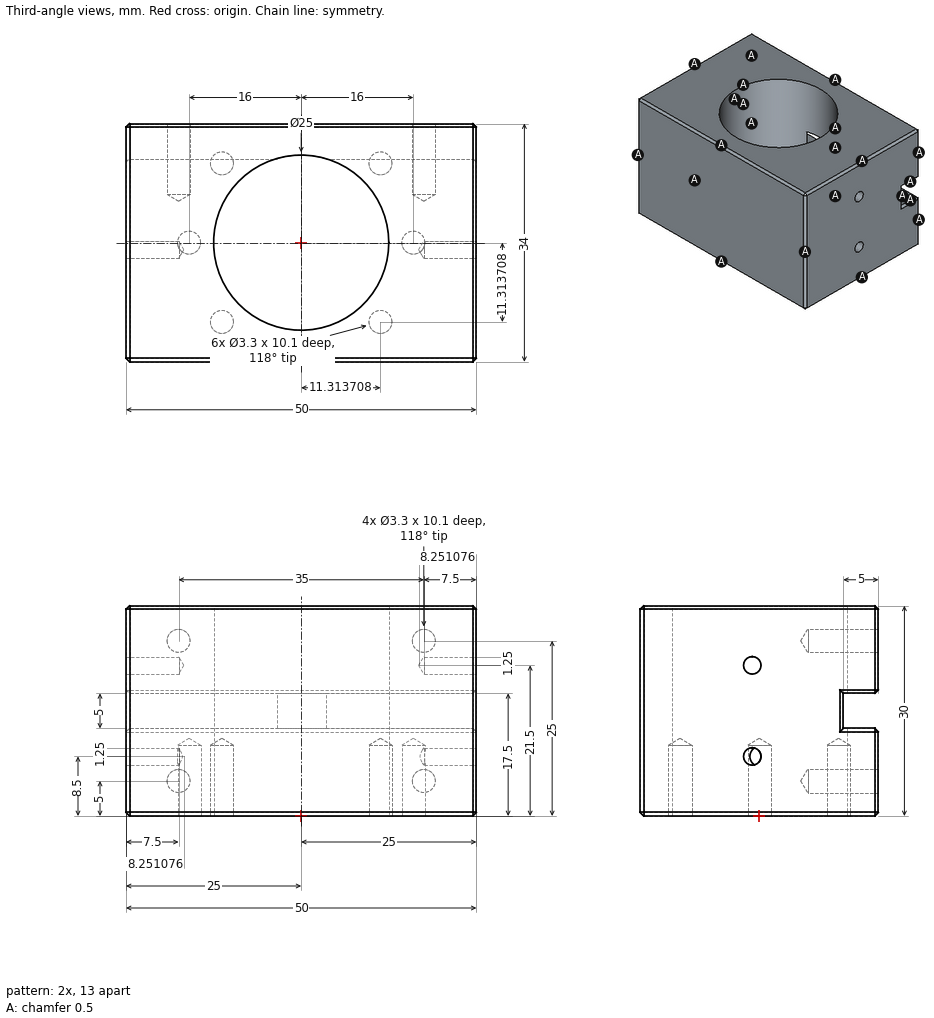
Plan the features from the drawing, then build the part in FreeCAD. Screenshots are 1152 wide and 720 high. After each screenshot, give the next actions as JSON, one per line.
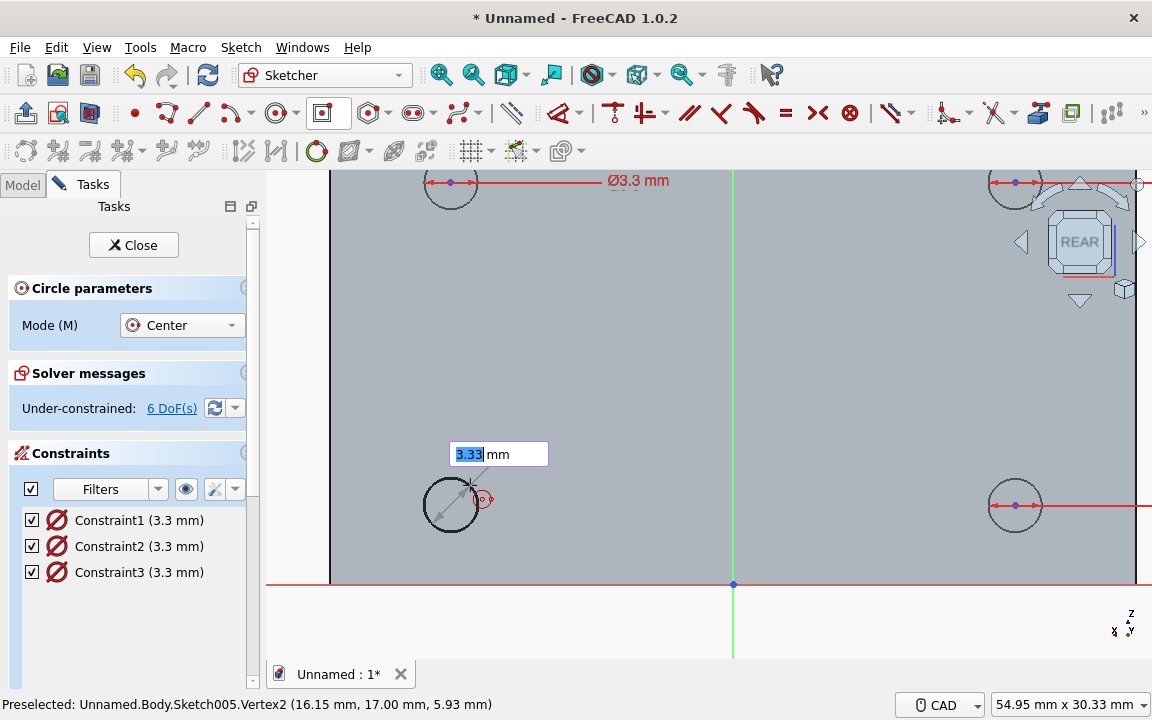
{"action": "type", "text": "3.3"}
{"action": "key", "text": "Return"}
{"action": "key", "text": "Escape"}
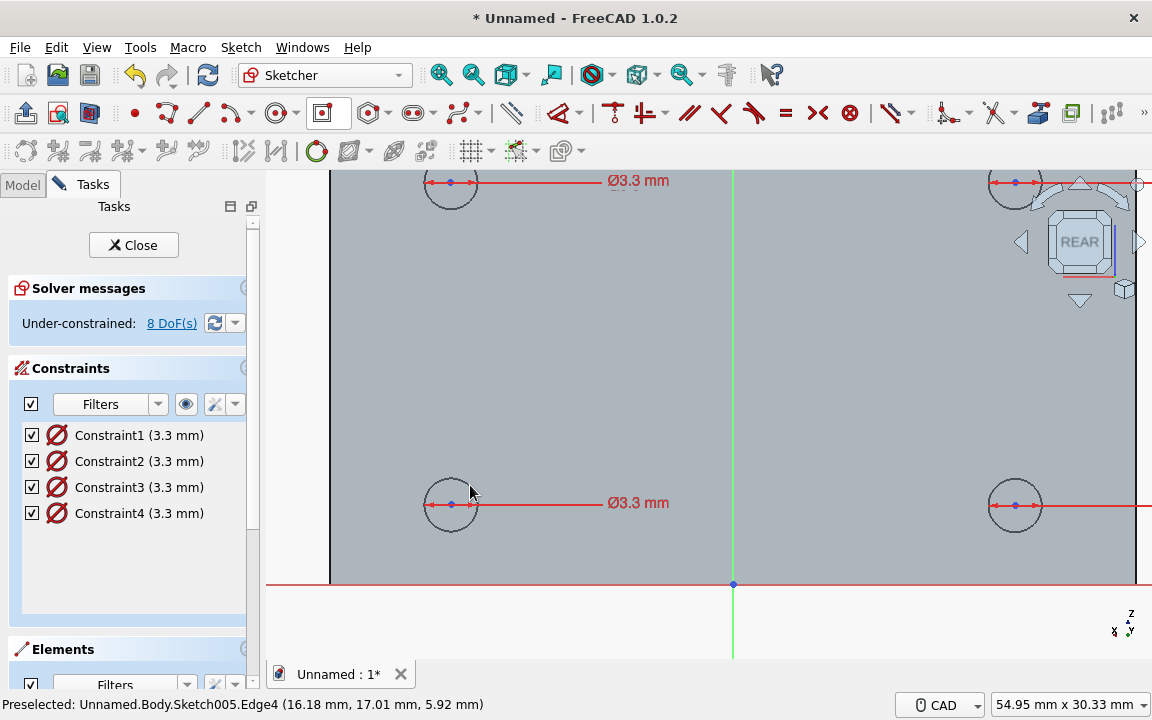
{"action": "scroll", "coordinate": [452, 505], "scroll_direction": "down", "scroll_amount": 2}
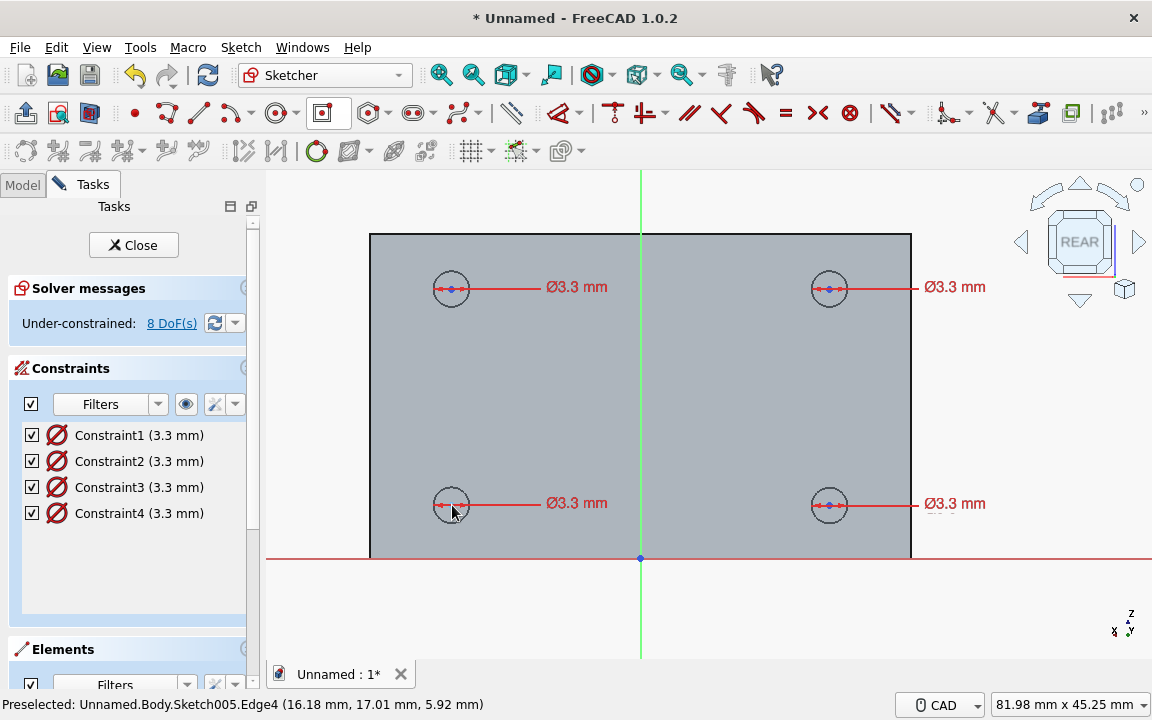
{"action": "left_click", "coordinate": [451, 289]}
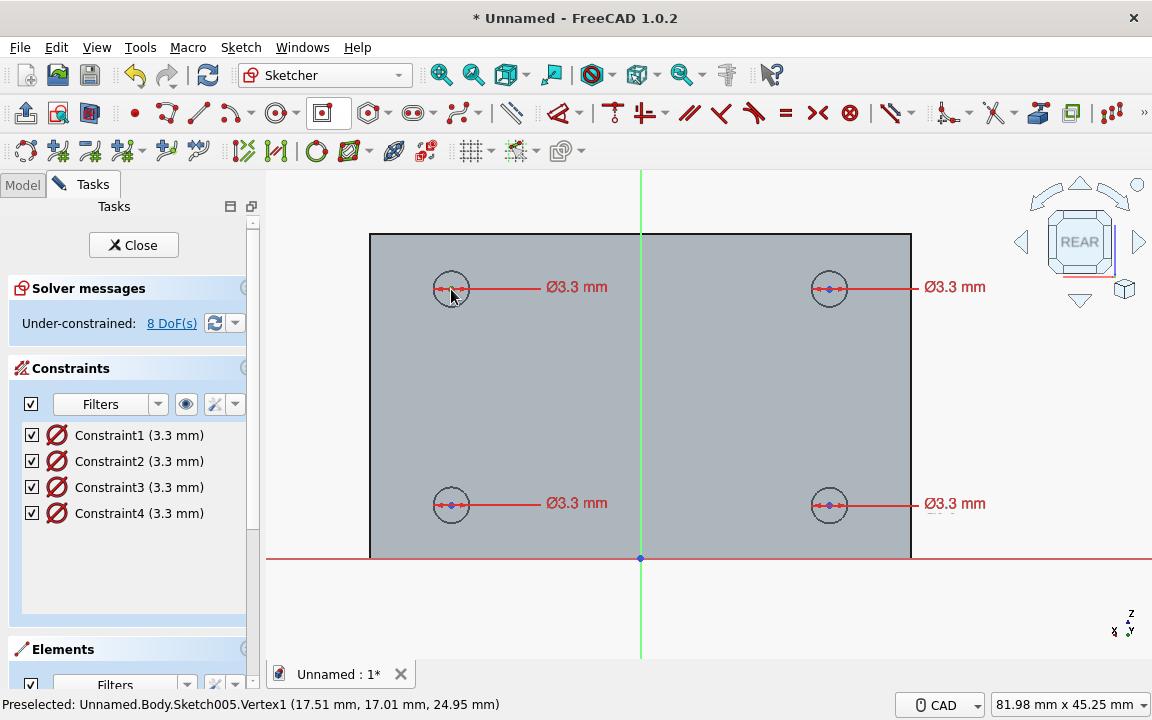
{"action": "left_click", "coordinate": [830, 289]}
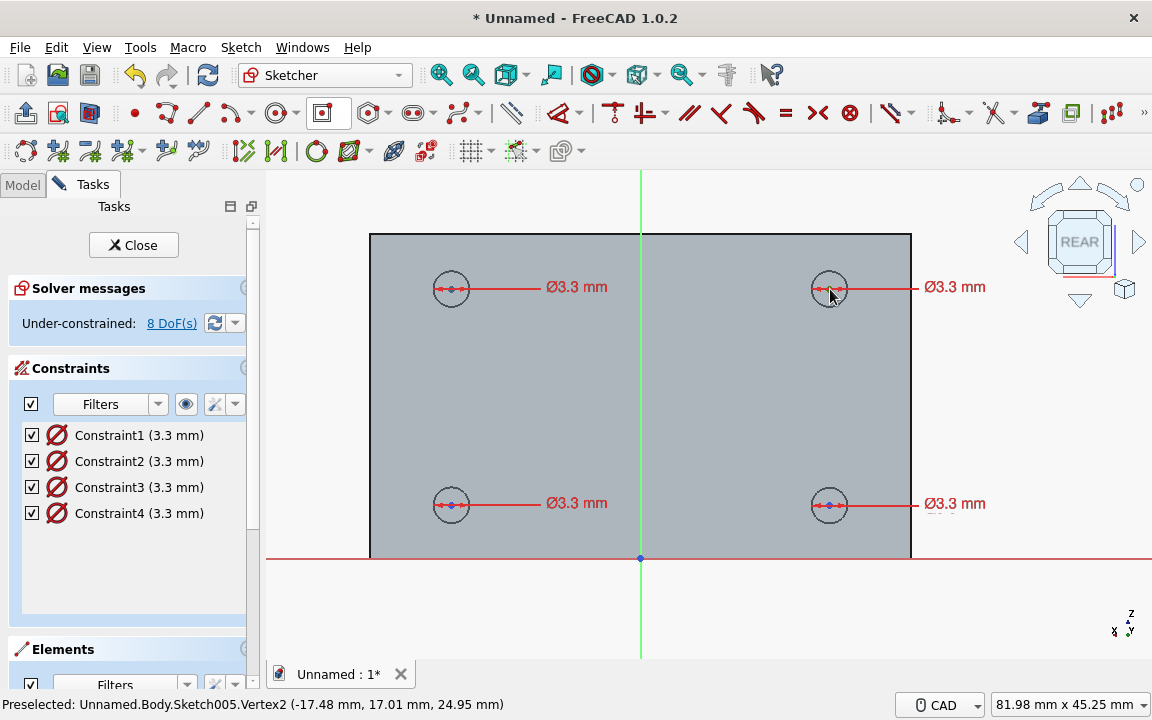
{"action": "left_click", "coordinate": [641, 600]}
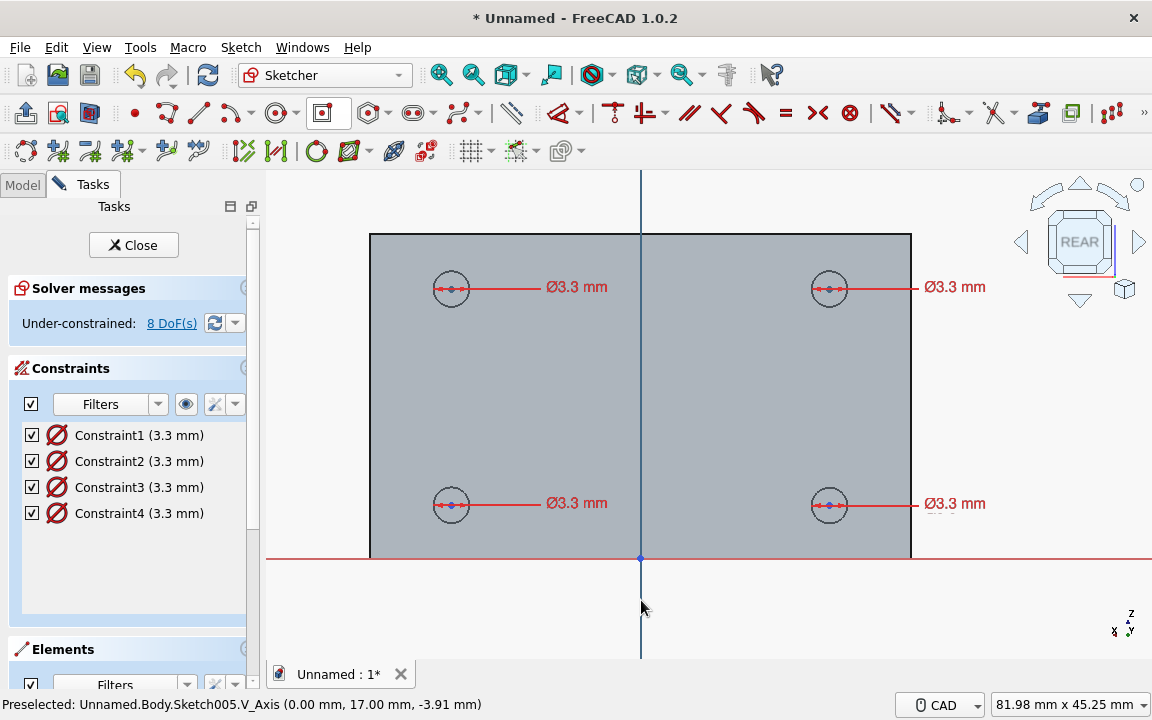
{"action": "key", "text": "s"}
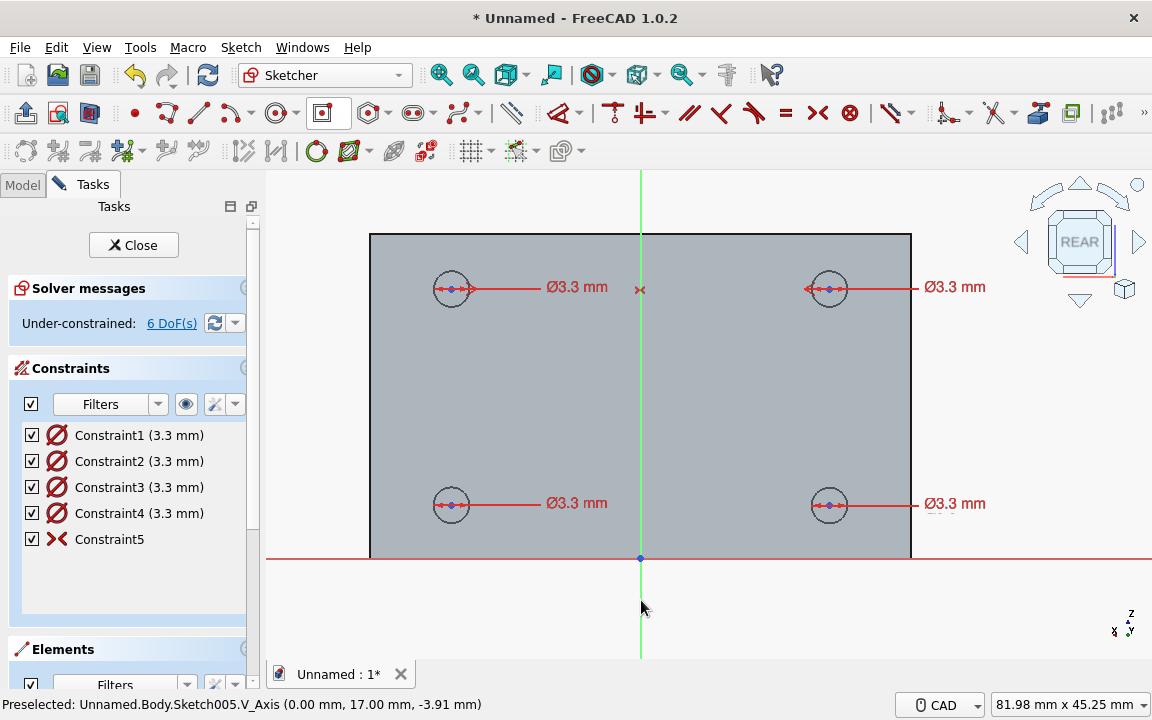
{"action": "left_click", "coordinate": [830, 506]}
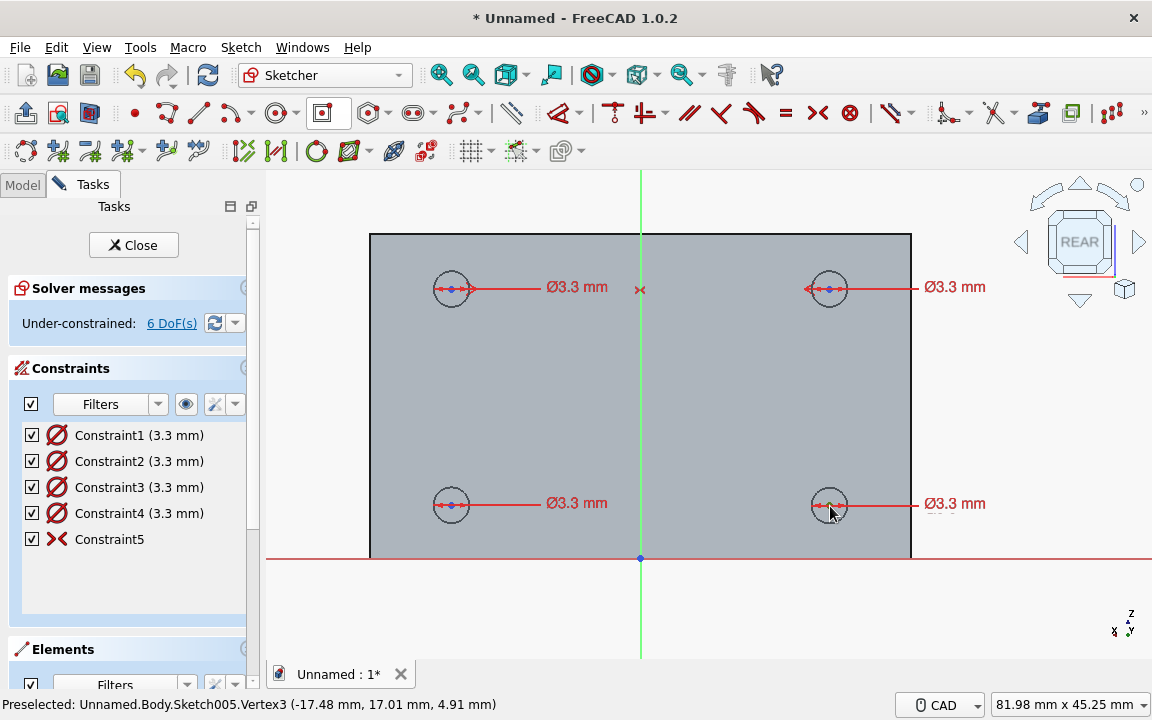
{"action": "left_click", "coordinate": [451, 505]}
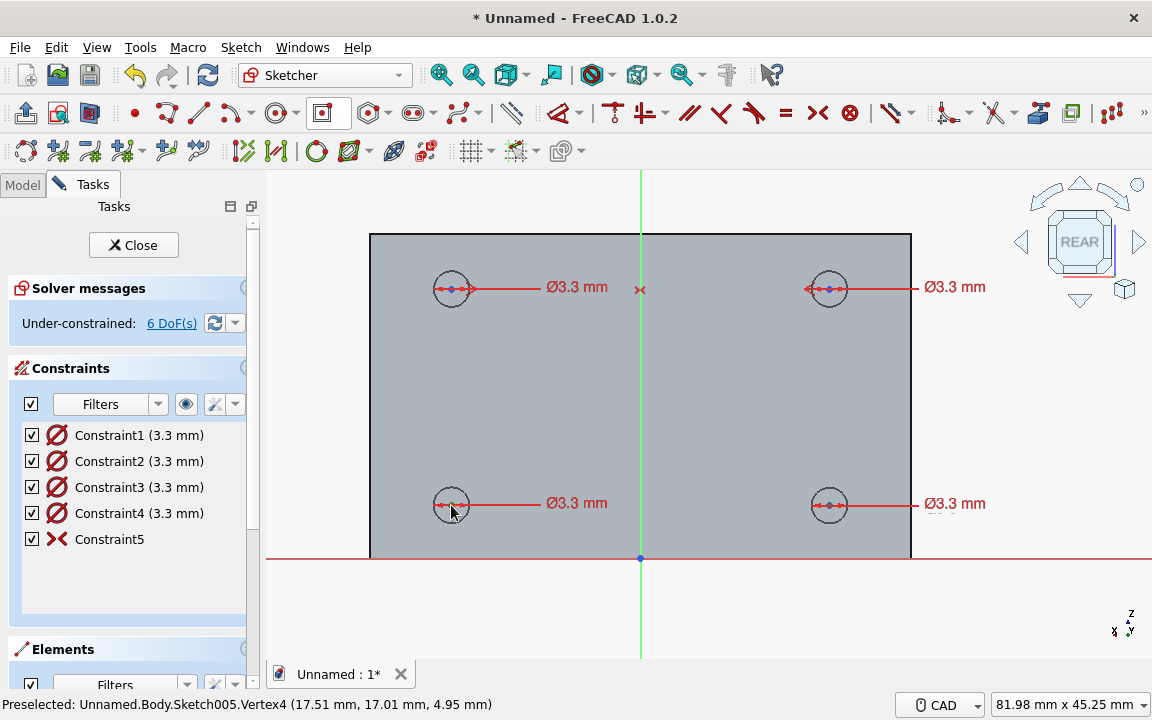
{"action": "left_click", "coordinate": [641, 600]}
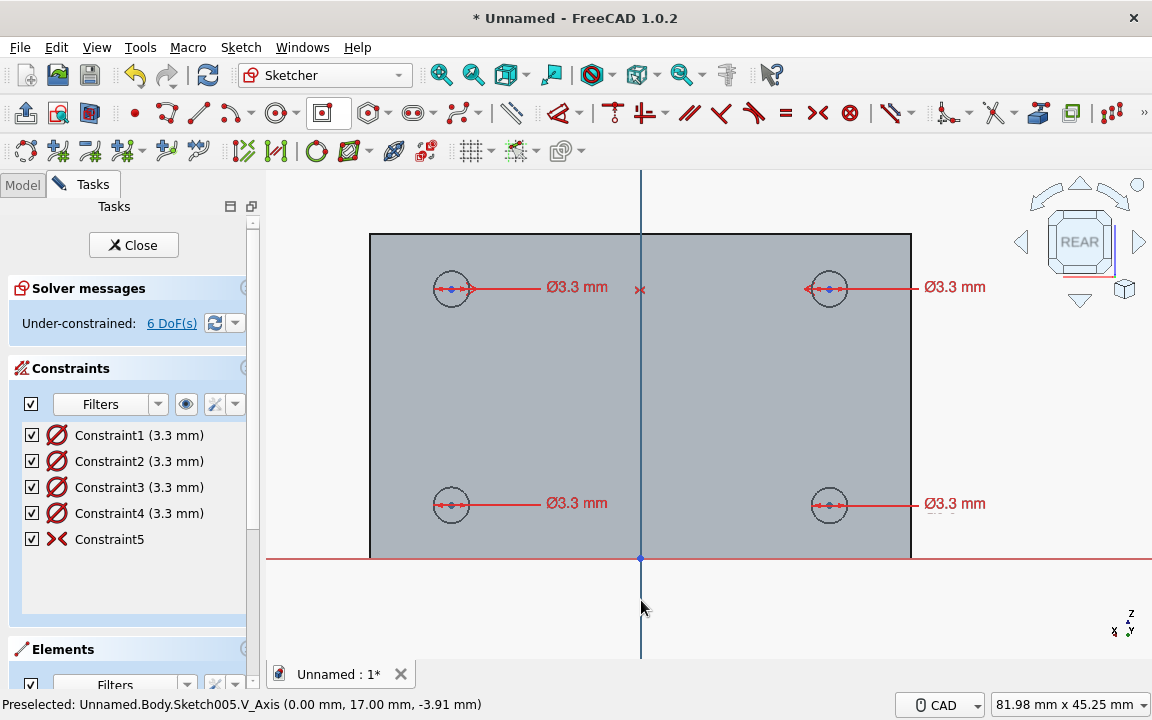
{"action": "key", "text": "s"}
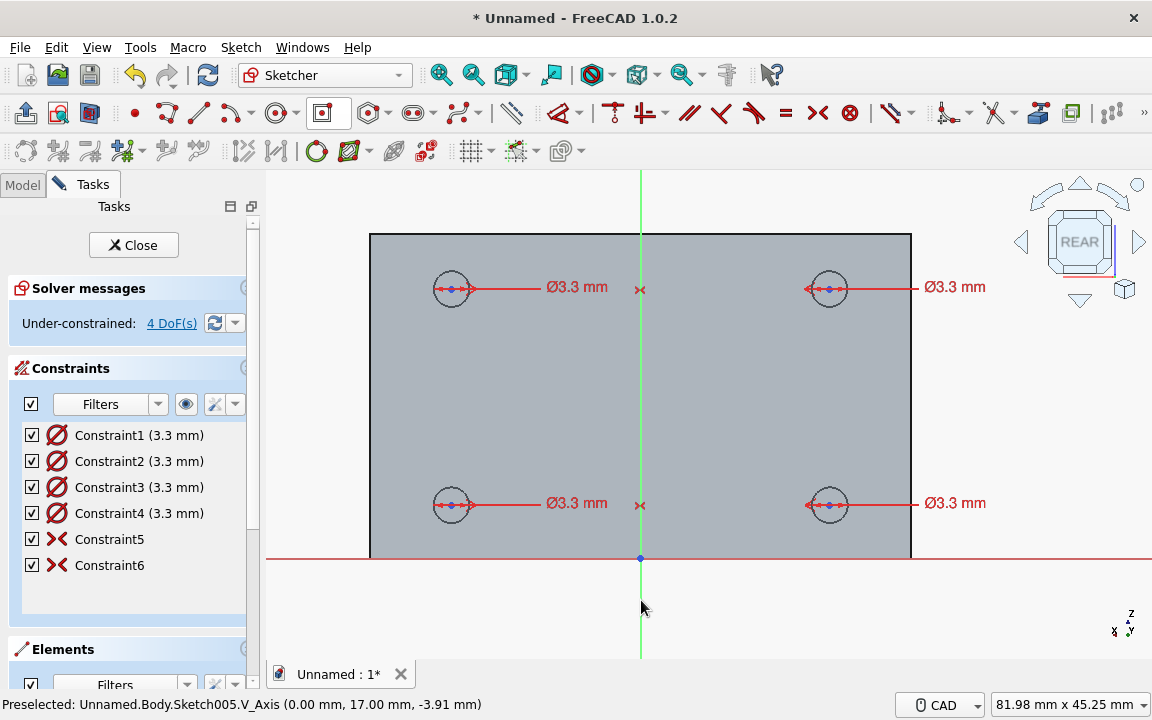
{"action": "left_click", "coordinate": [558, 114]}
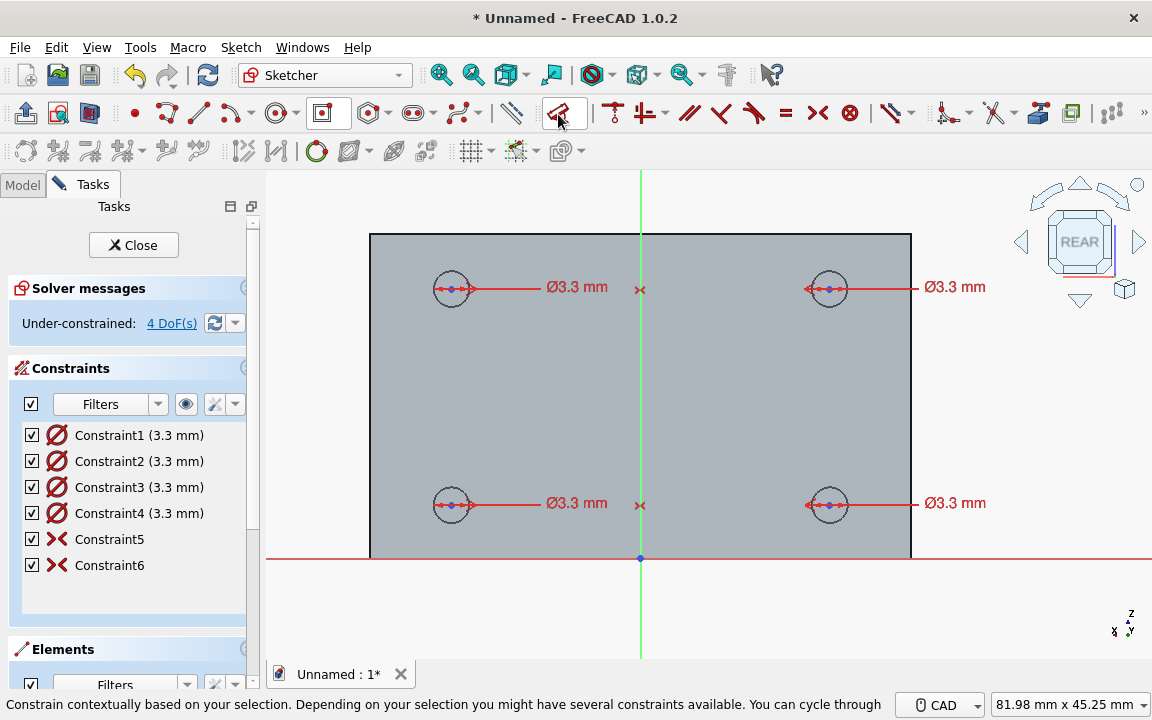
{"action": "left_click", "coordinate": [830, 505]}
{"action": "left_click", "coordinate": [864, 532]}